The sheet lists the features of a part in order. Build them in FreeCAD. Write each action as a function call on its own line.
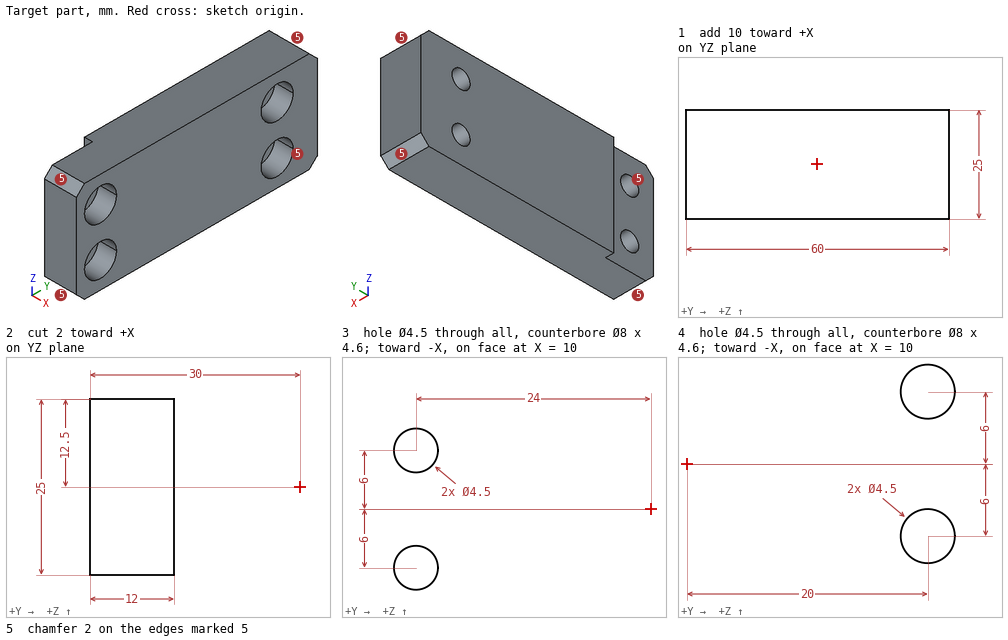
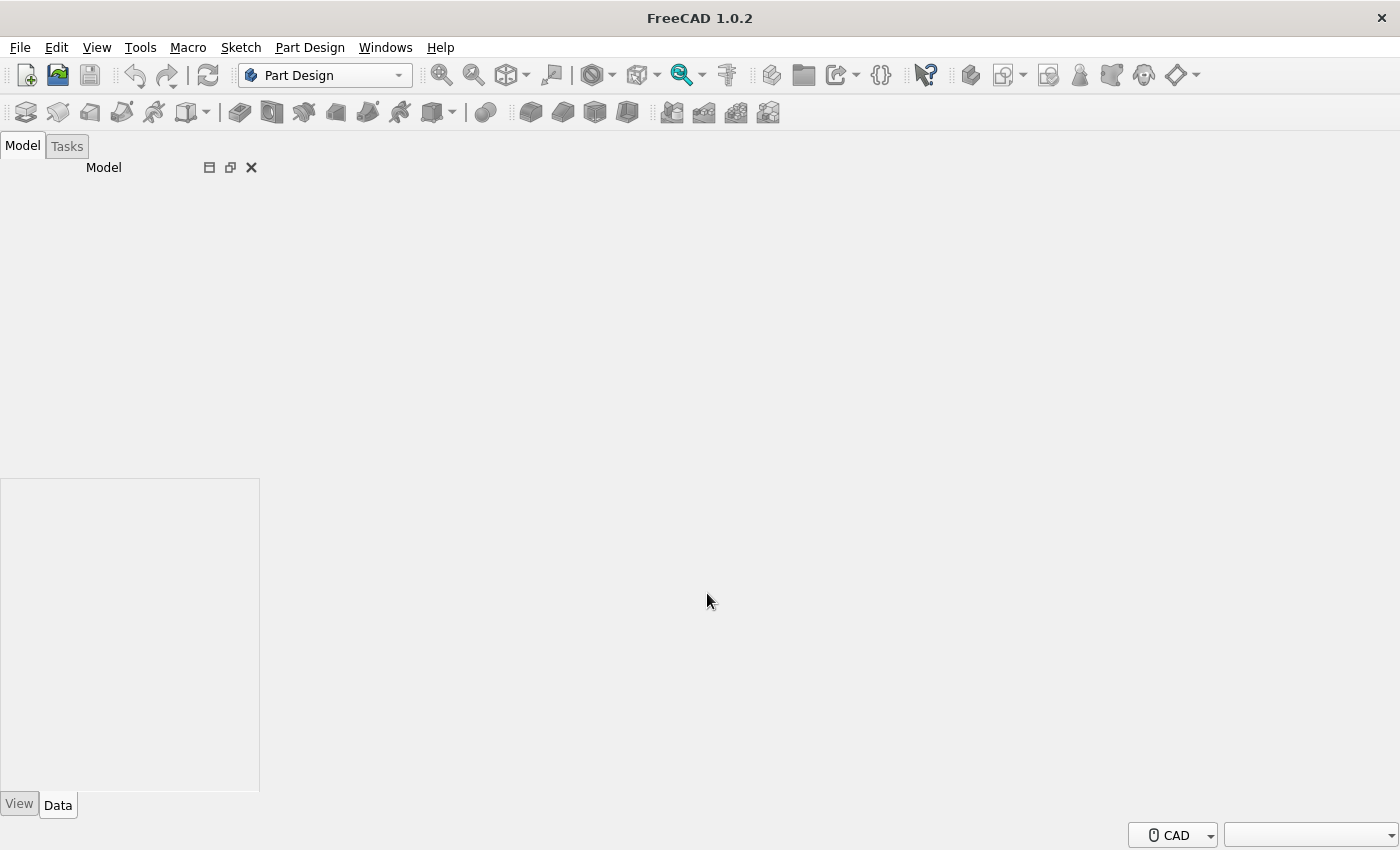
key(ctrl+n)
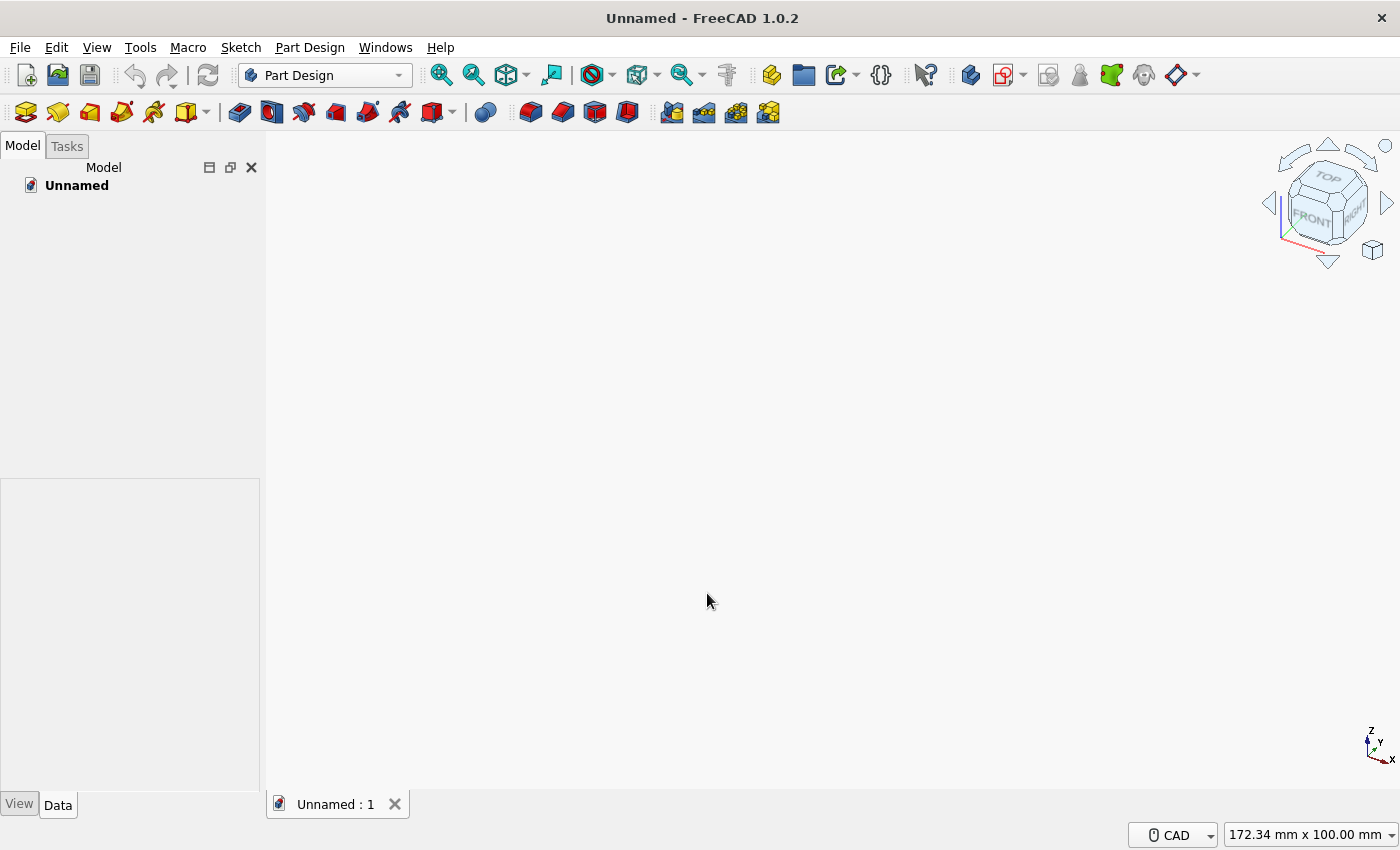
click(1004, 76)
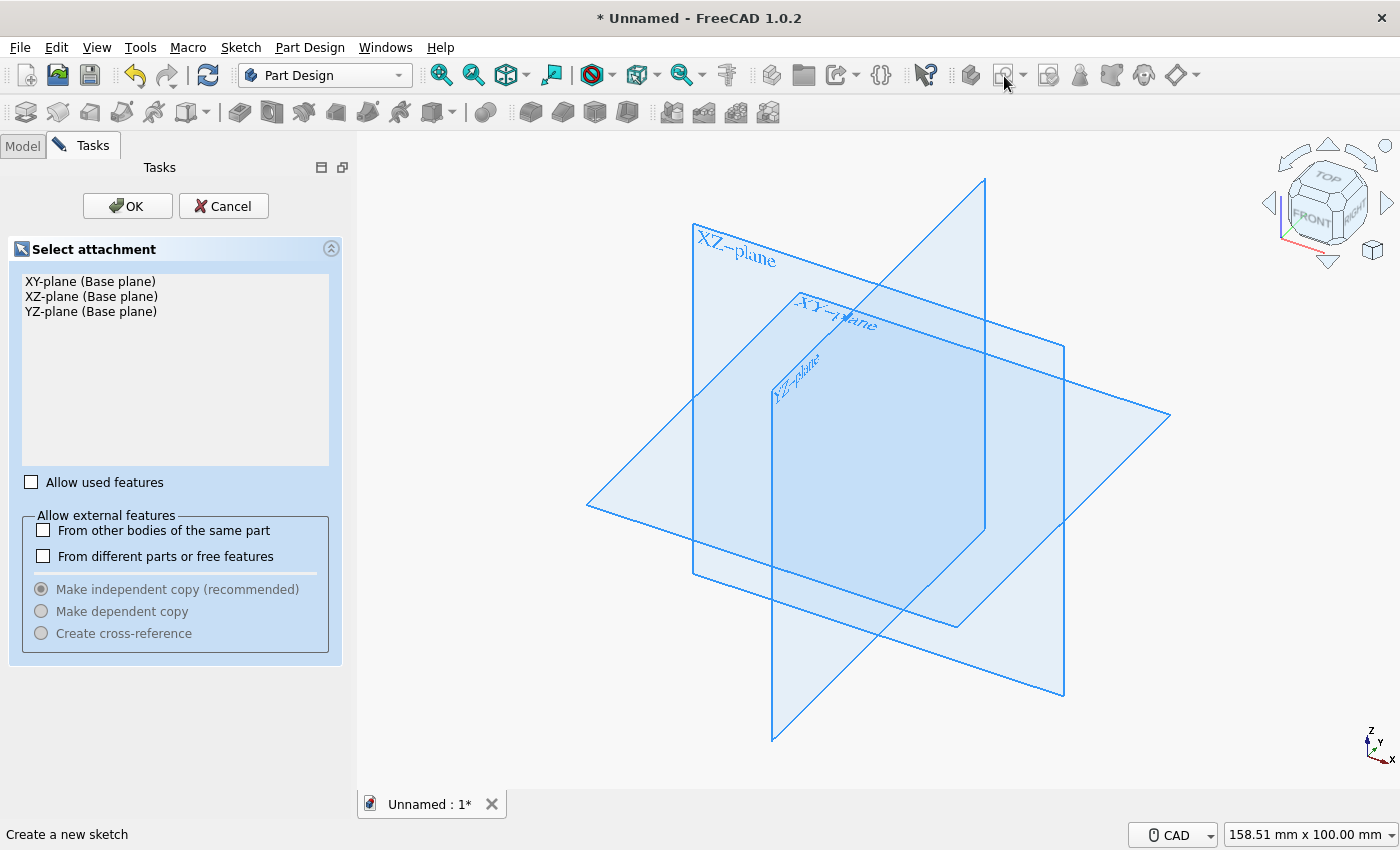
click(82, 312)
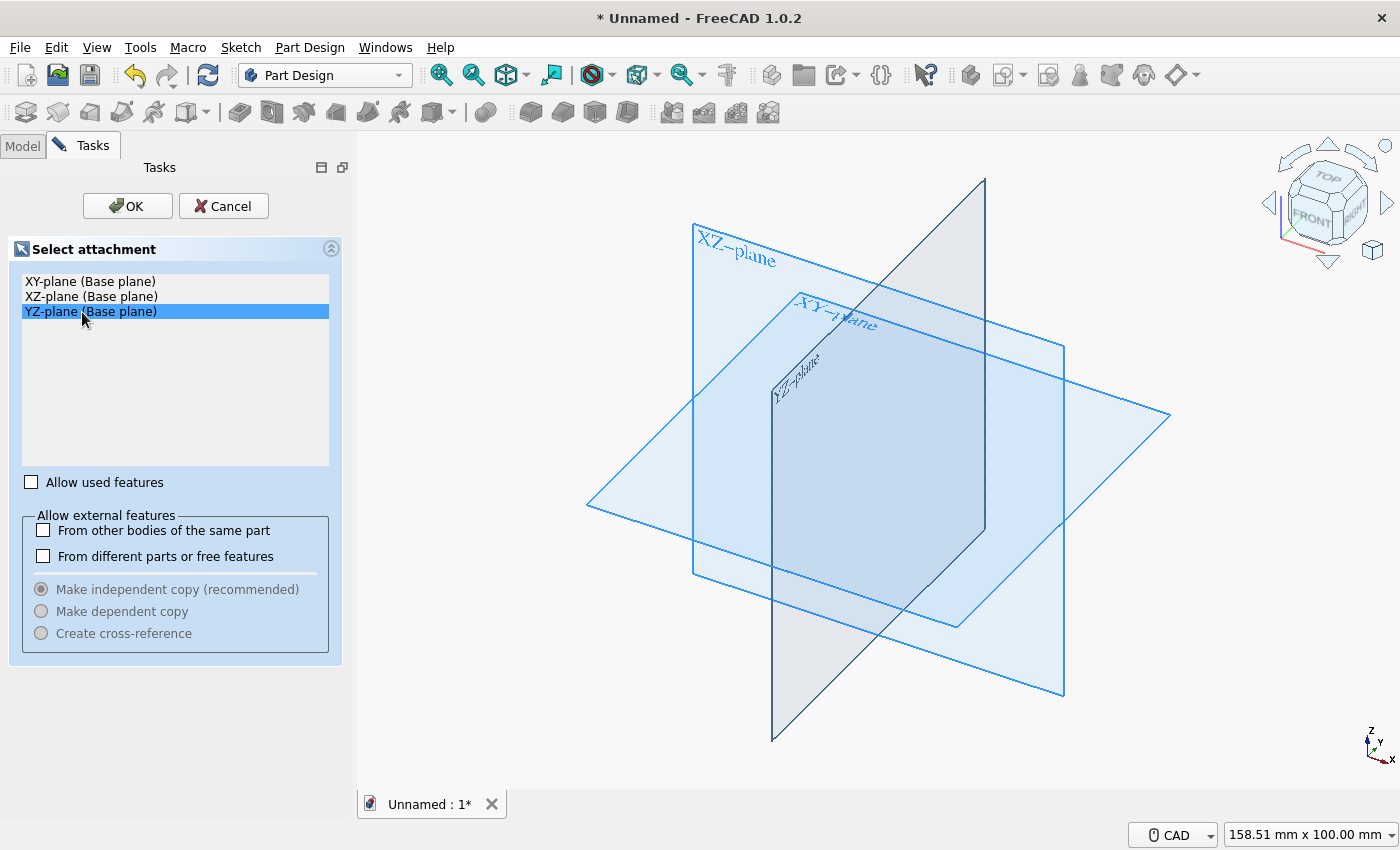
click(128, 206)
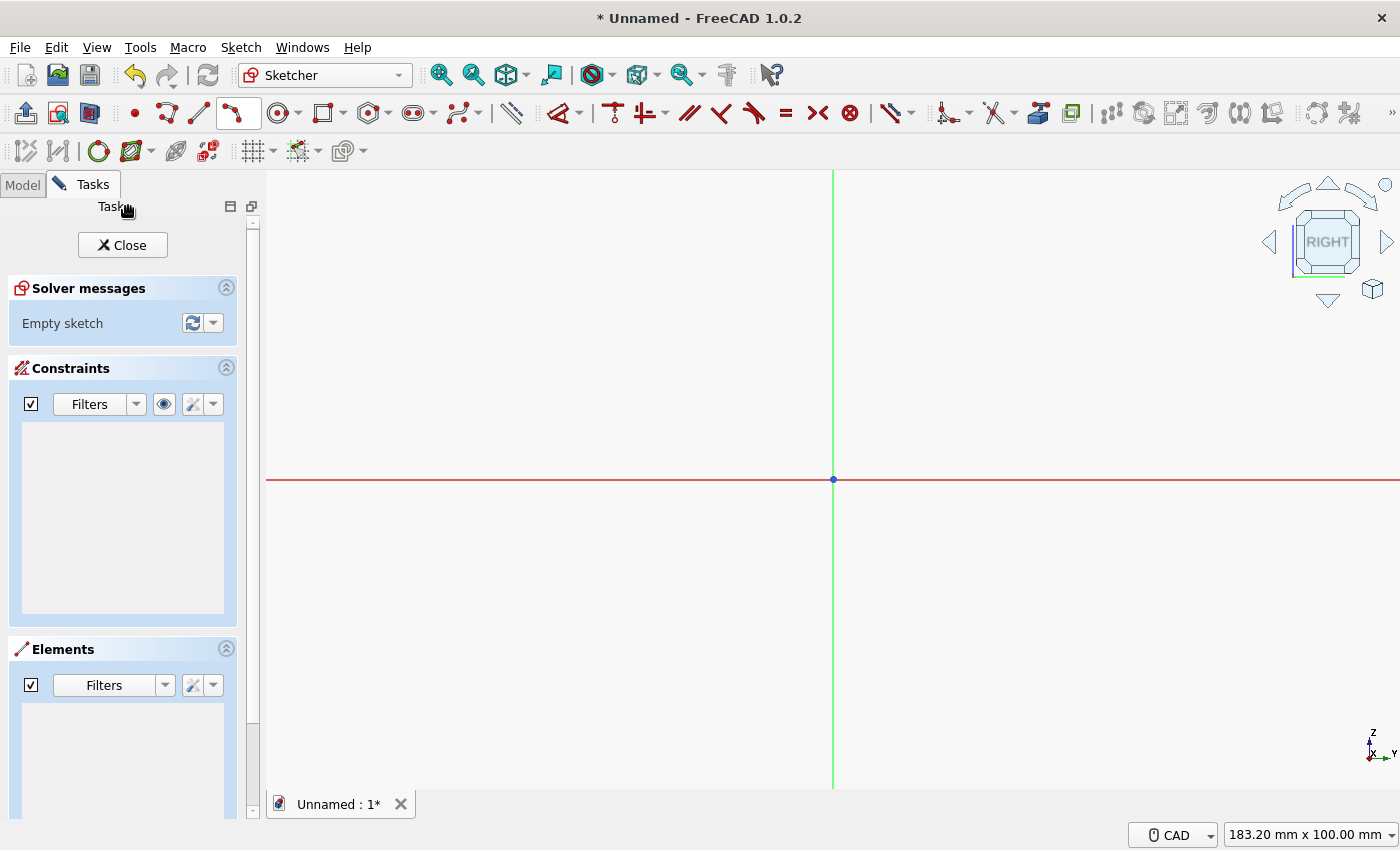
scroll(916, 480, up, 3)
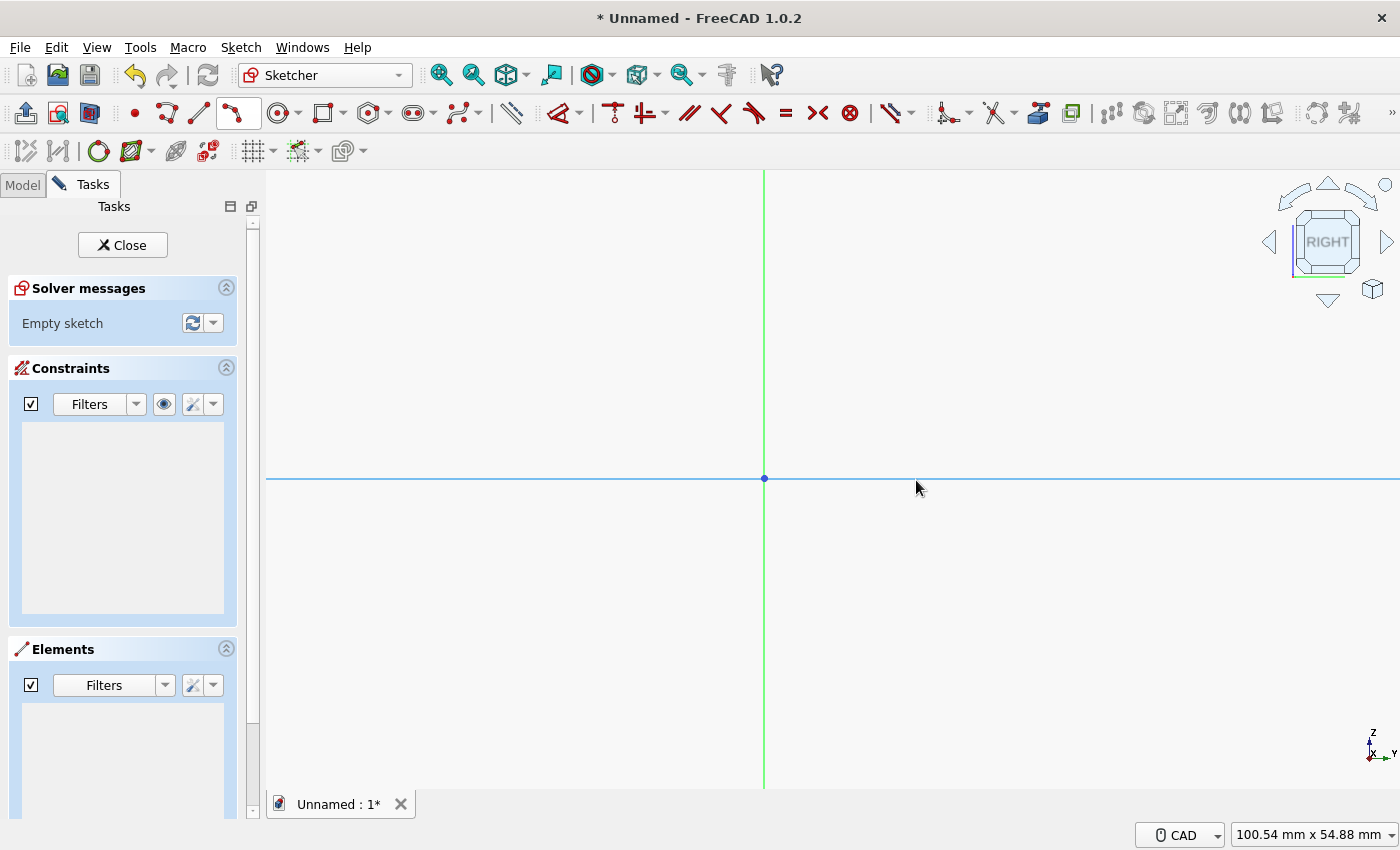
key(g)
key(v)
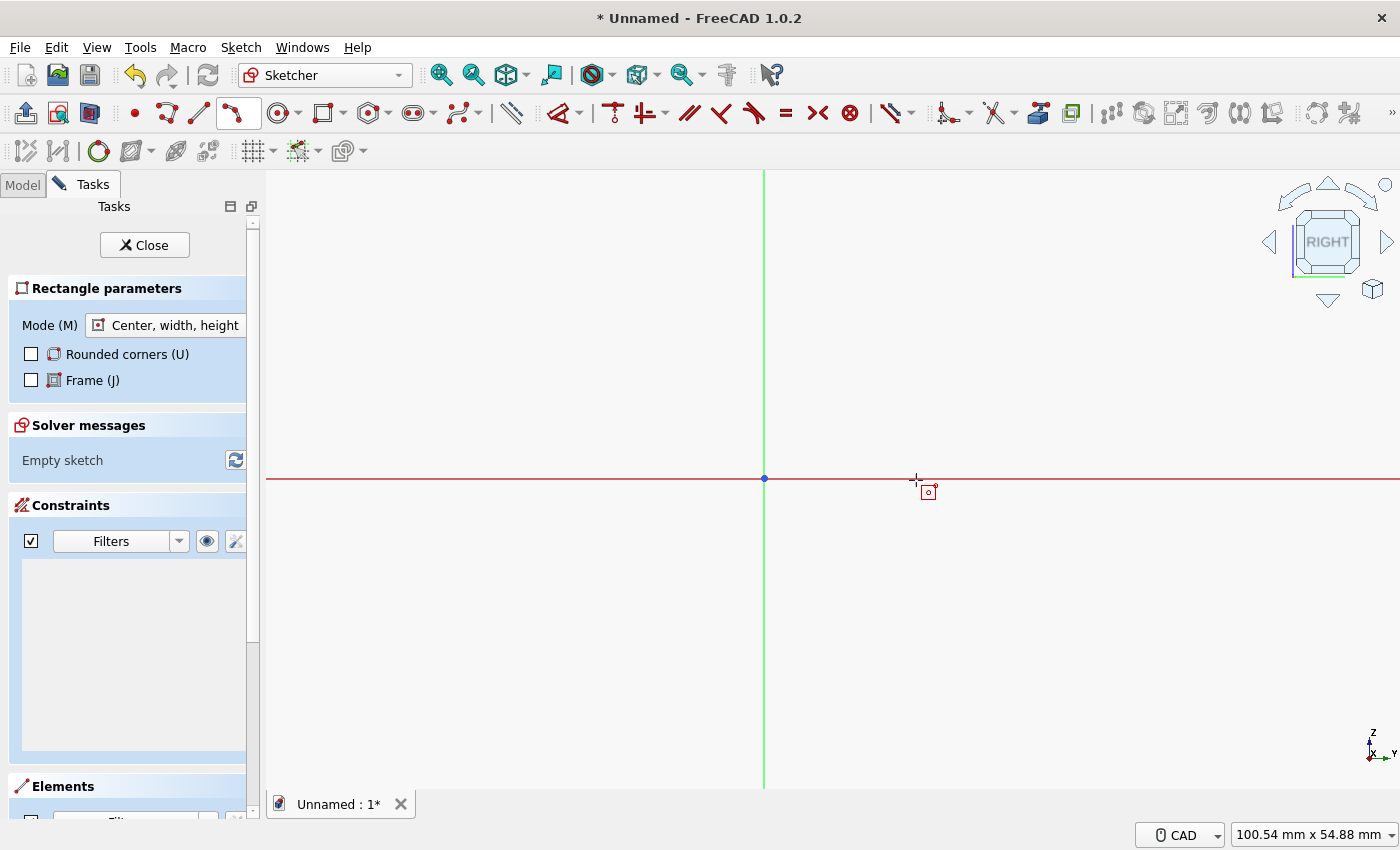
click(764, 479)
click(1103, 338)
key(Escape)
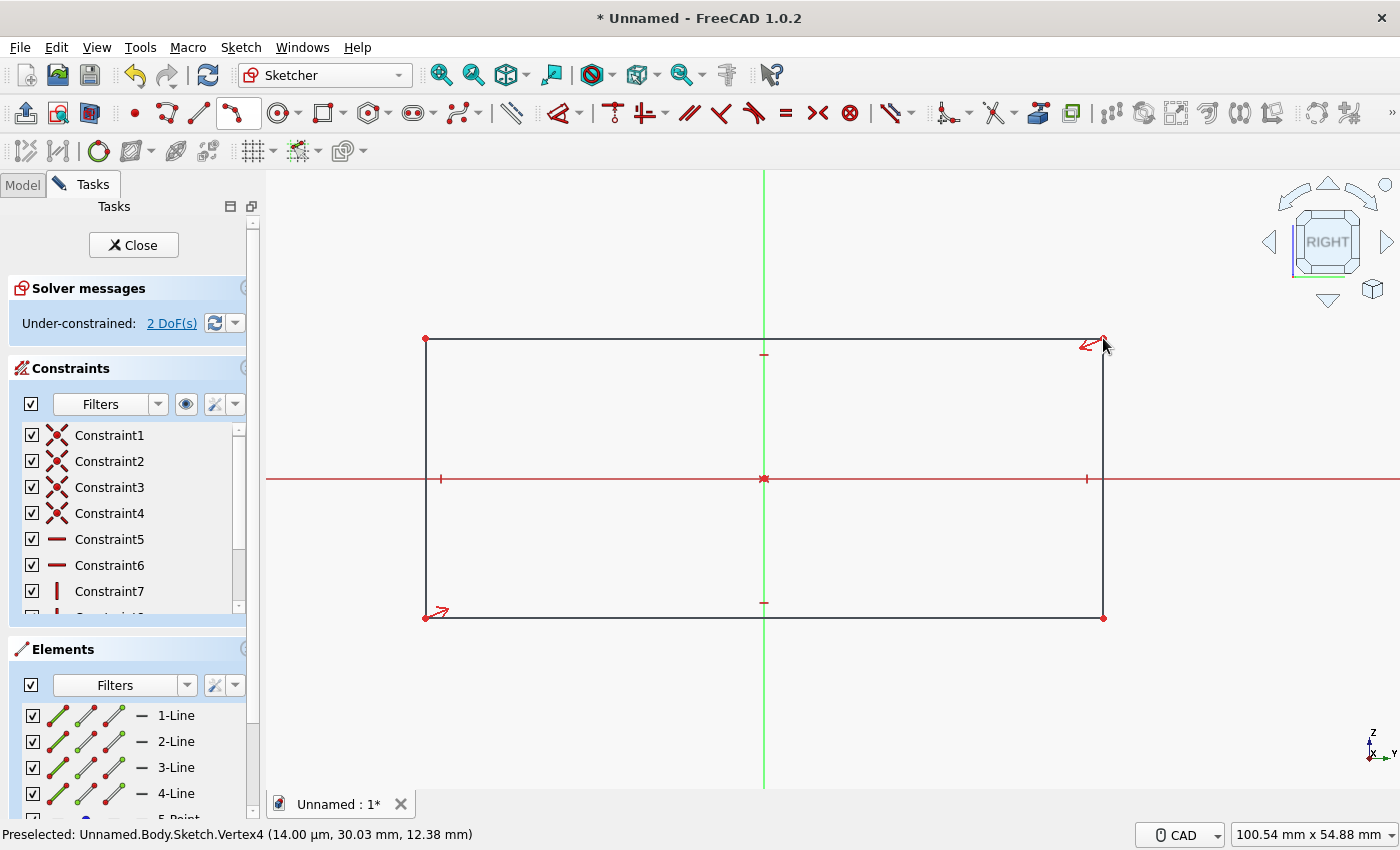
click(629, 618)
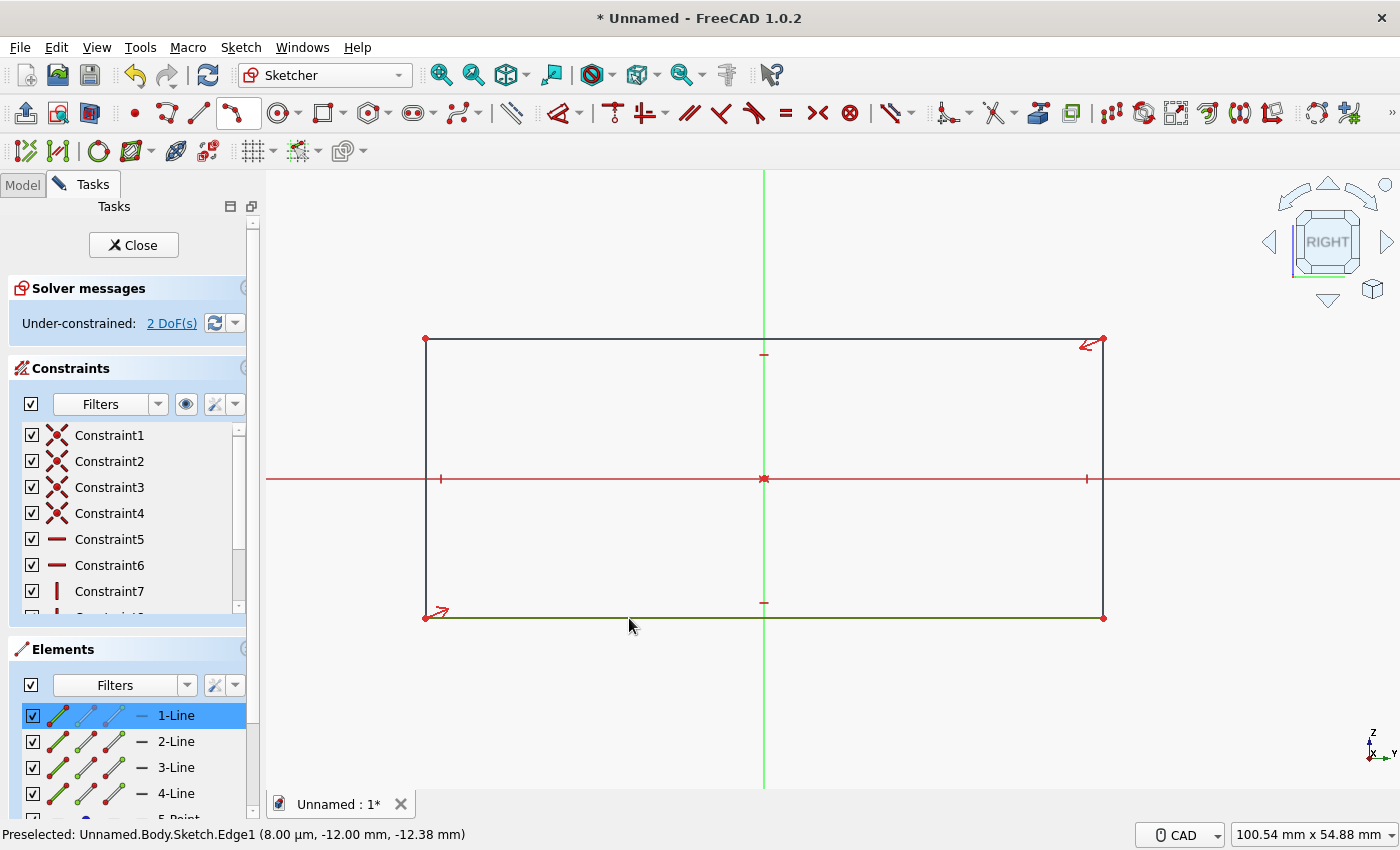
click(582, 114)